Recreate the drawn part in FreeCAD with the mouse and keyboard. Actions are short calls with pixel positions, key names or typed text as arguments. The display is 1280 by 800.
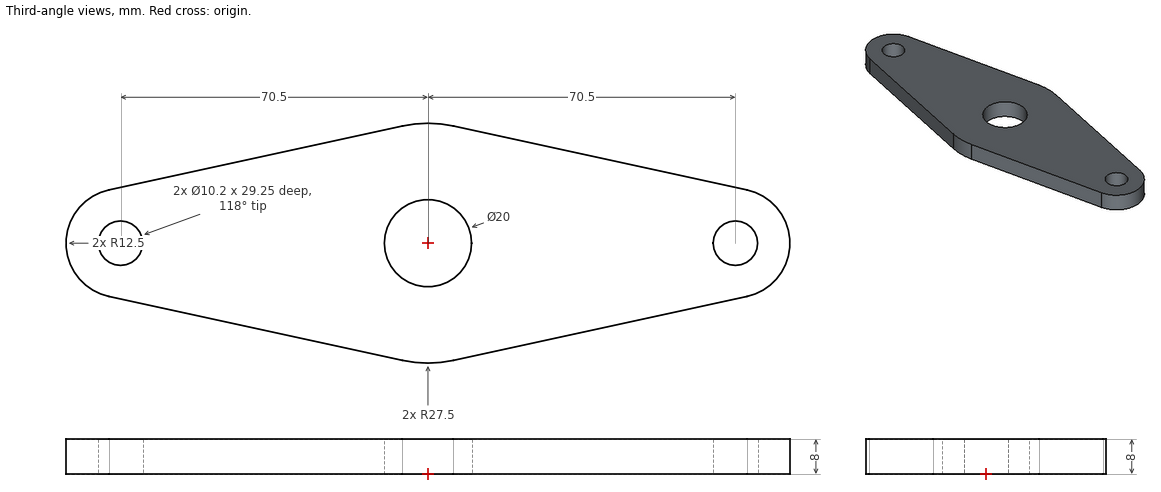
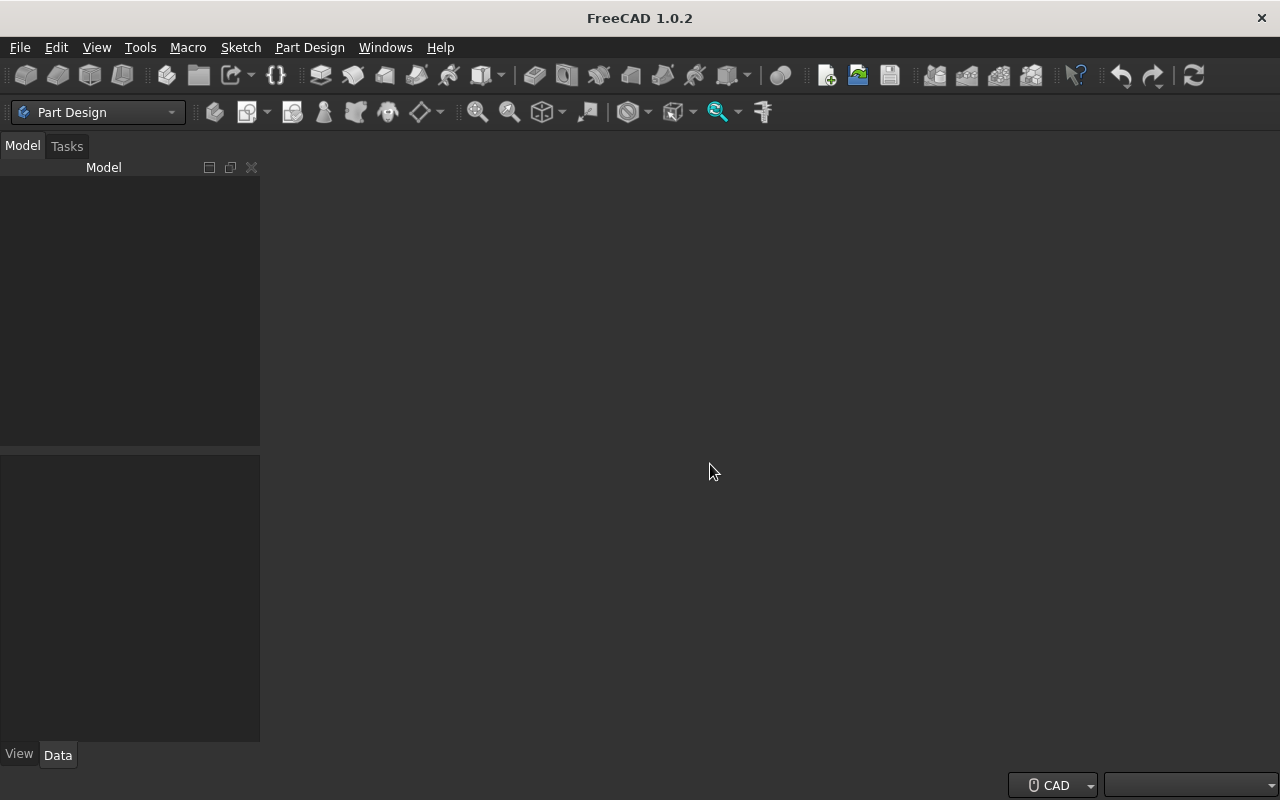
click(826, 76)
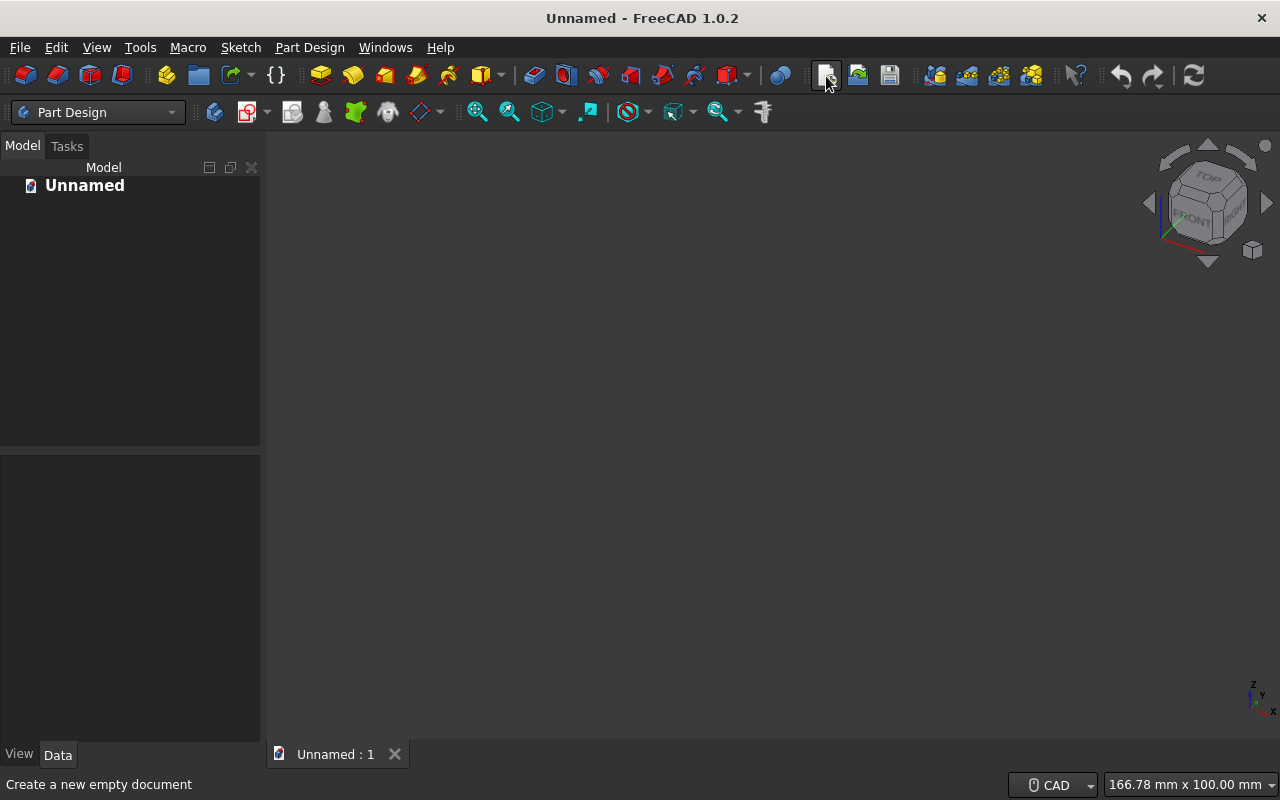
click(248, 112)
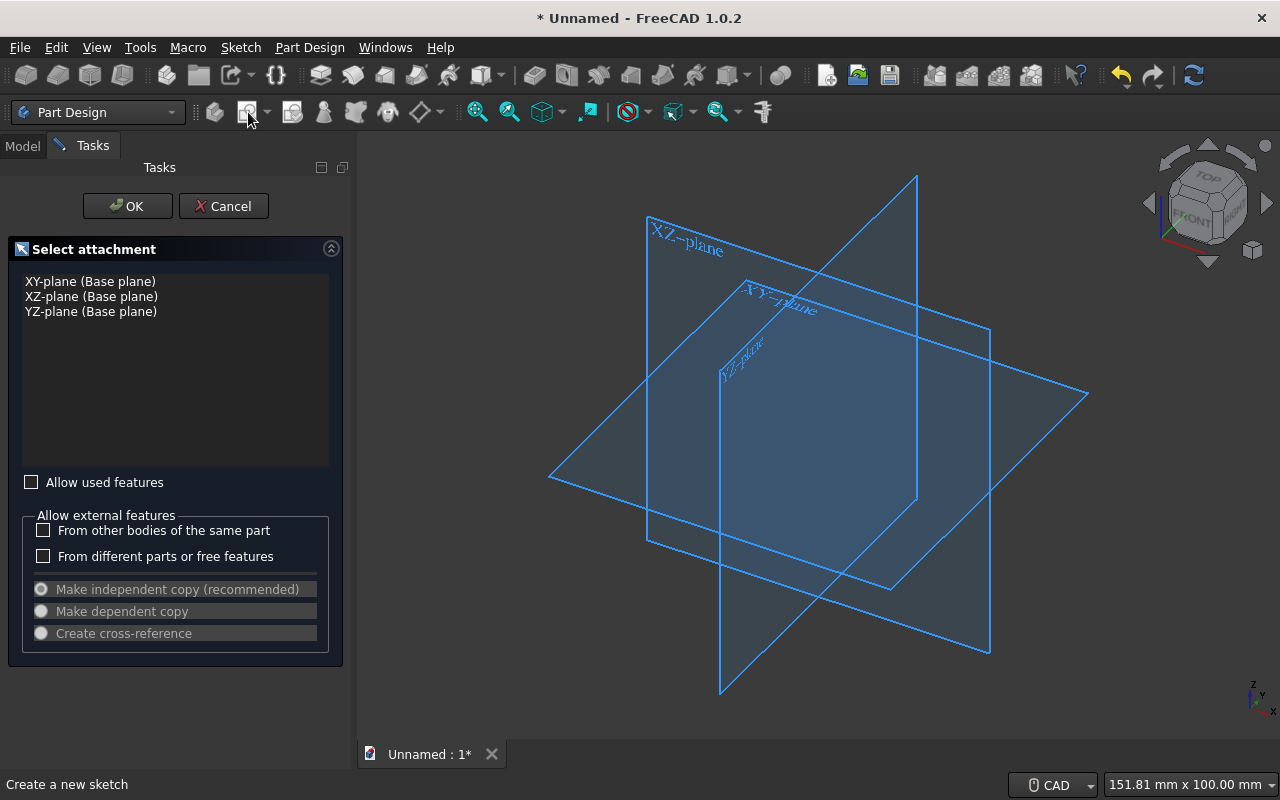
click(82, 282)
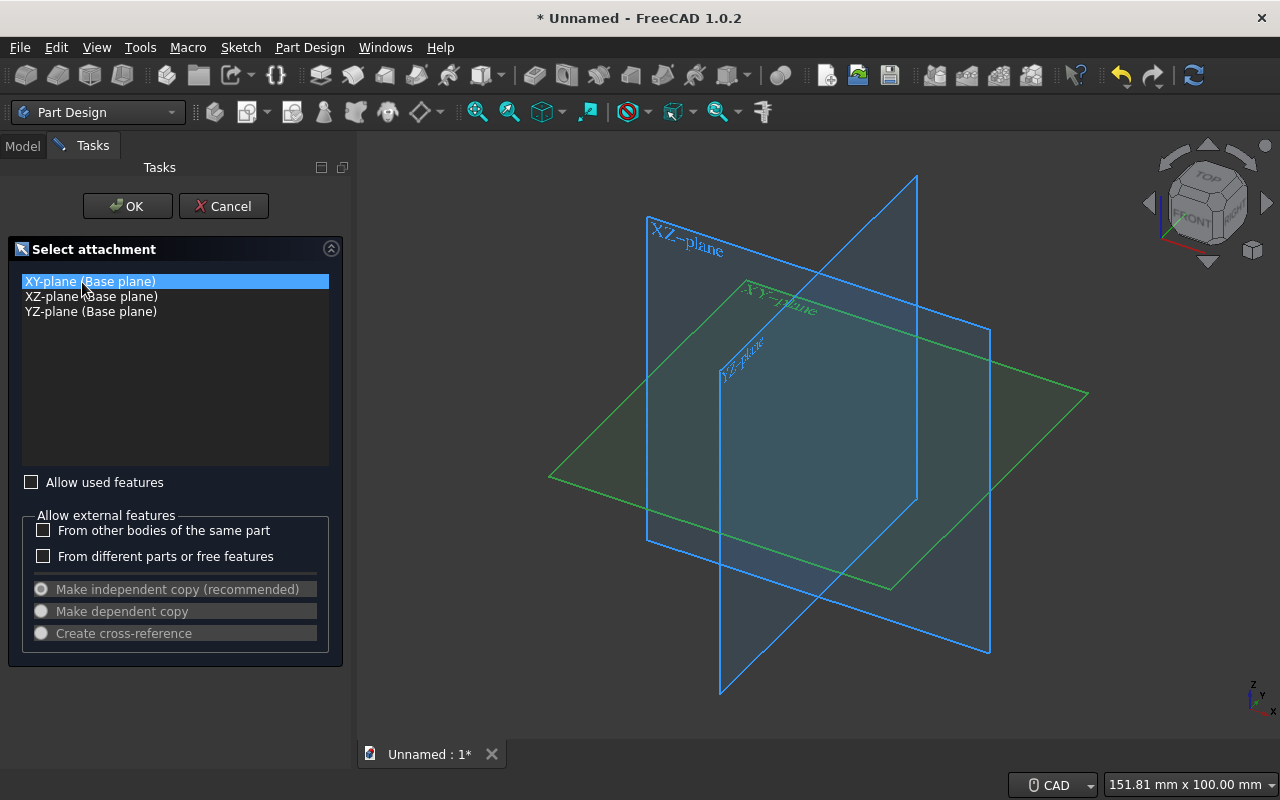
click(128, 206)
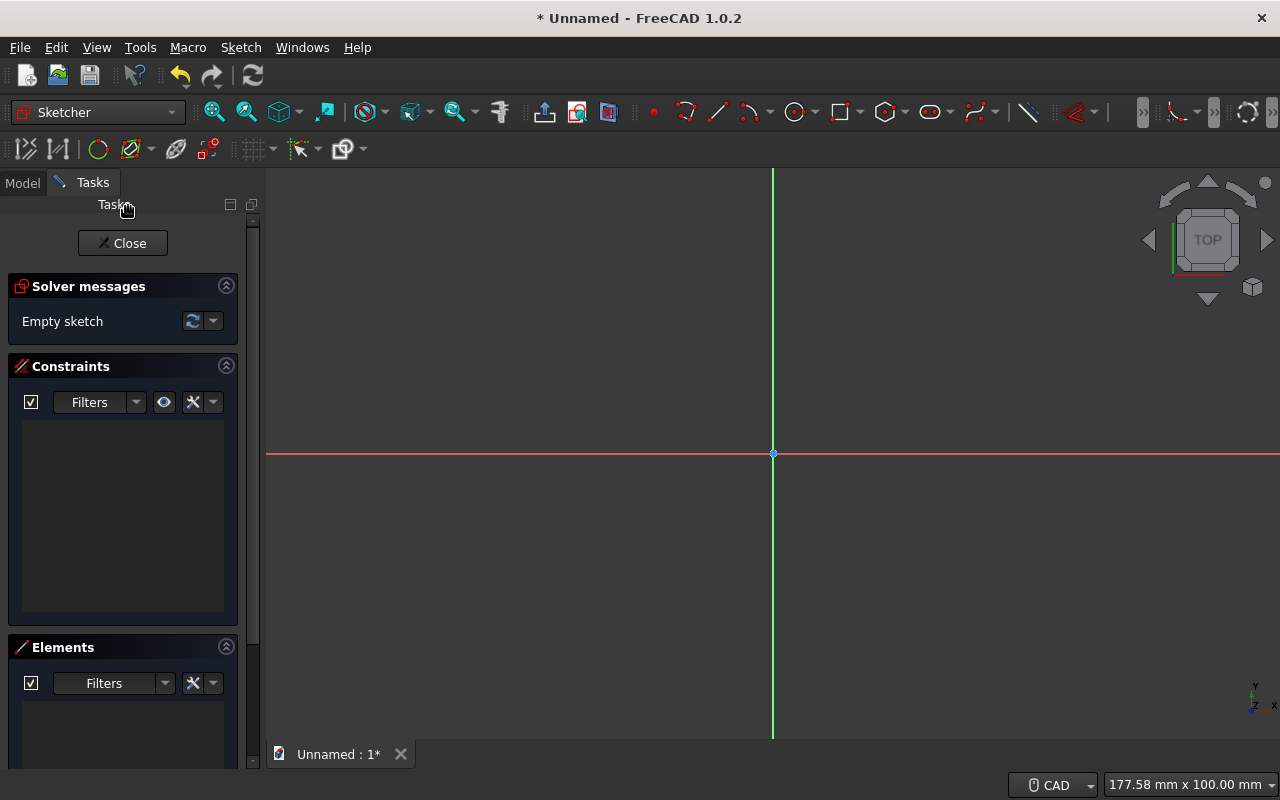
scroll(565, 453, down, 2)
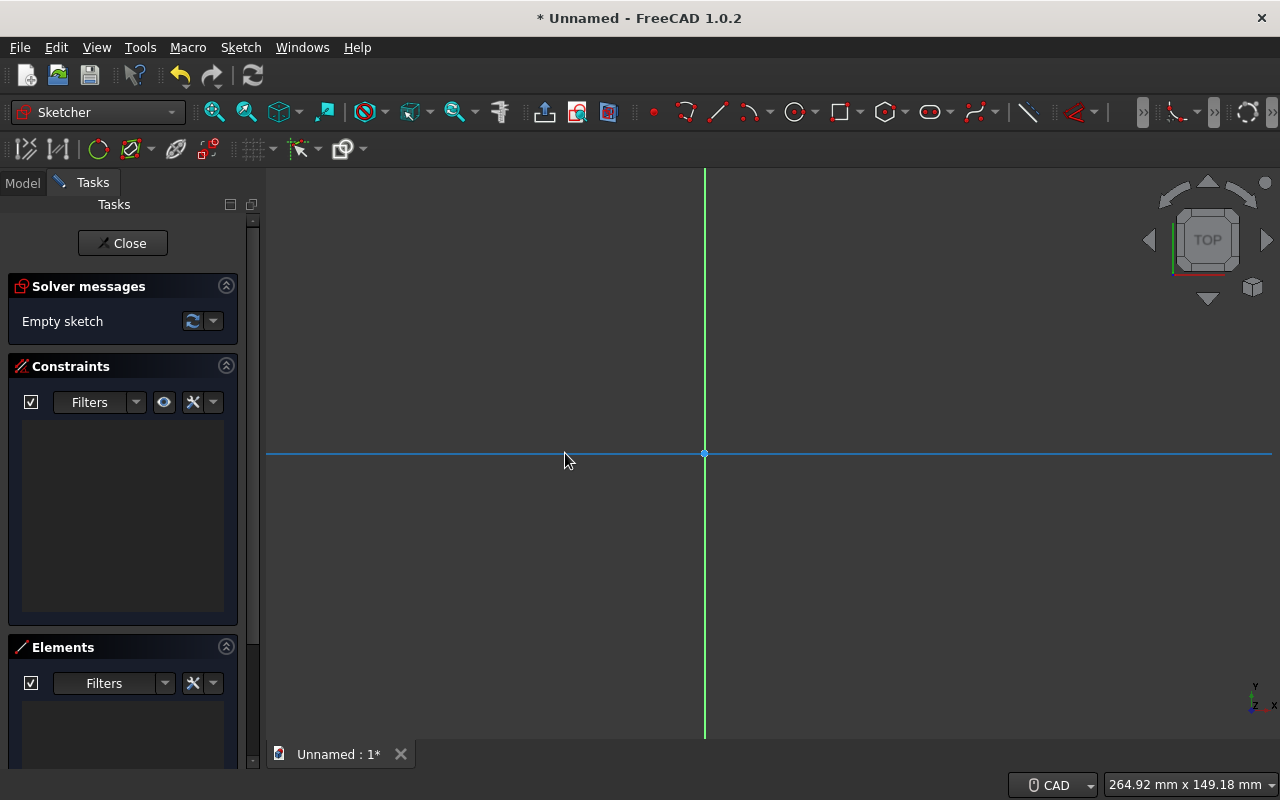
click(718, 112)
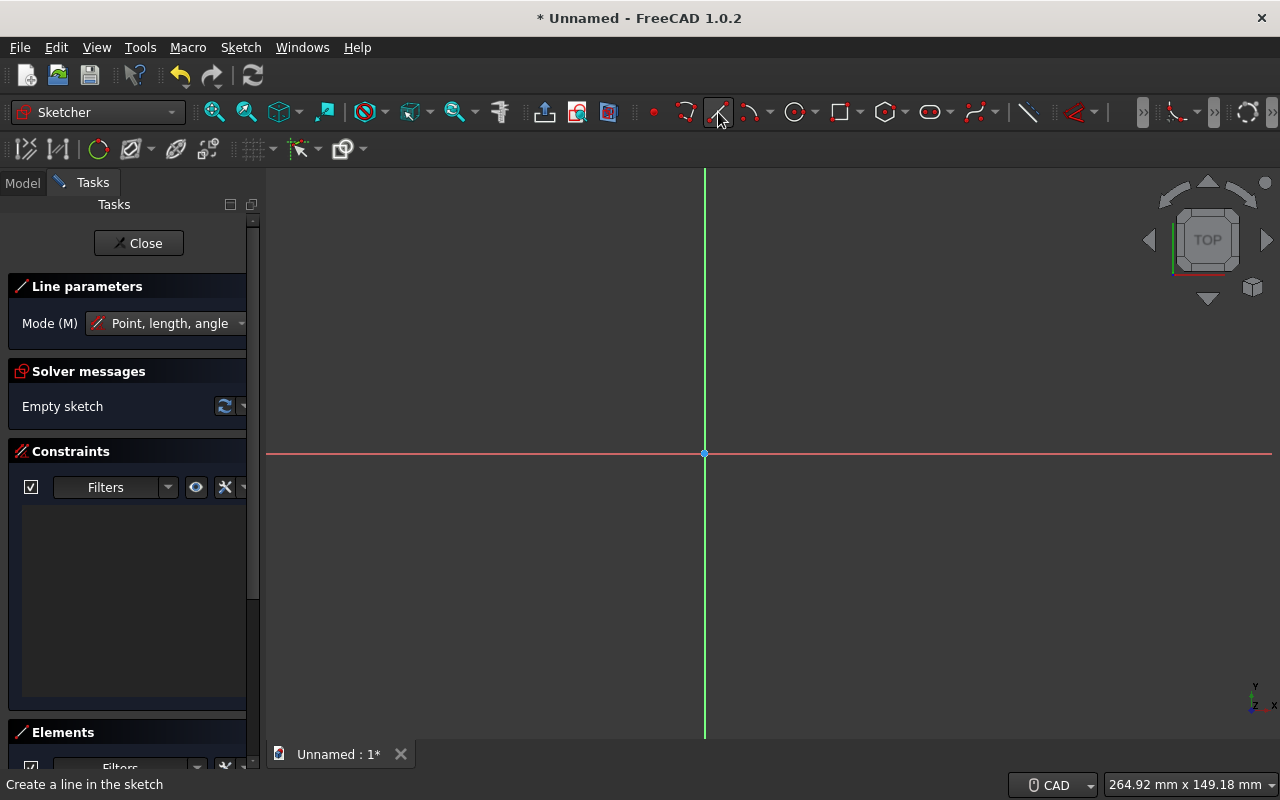
click(682, 351)
click(425, 407)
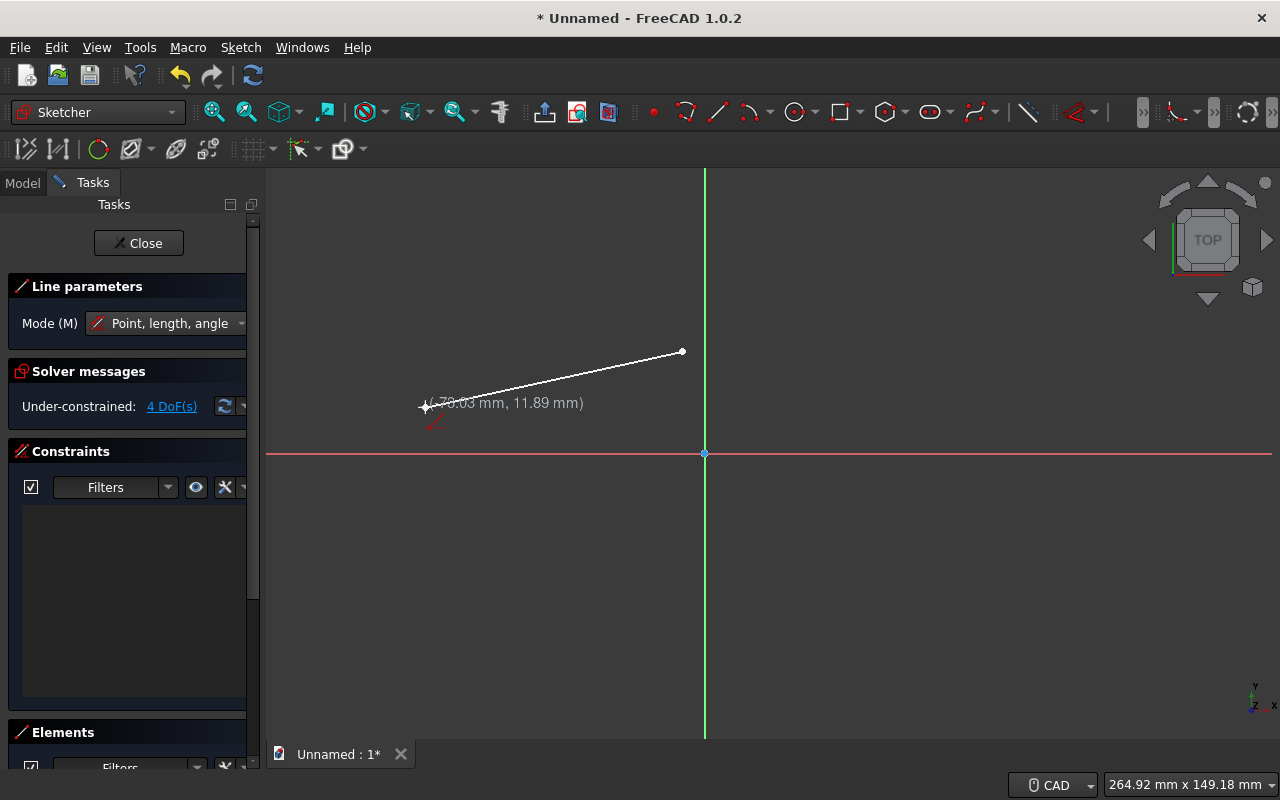
click(425, 500)
click(682, 556)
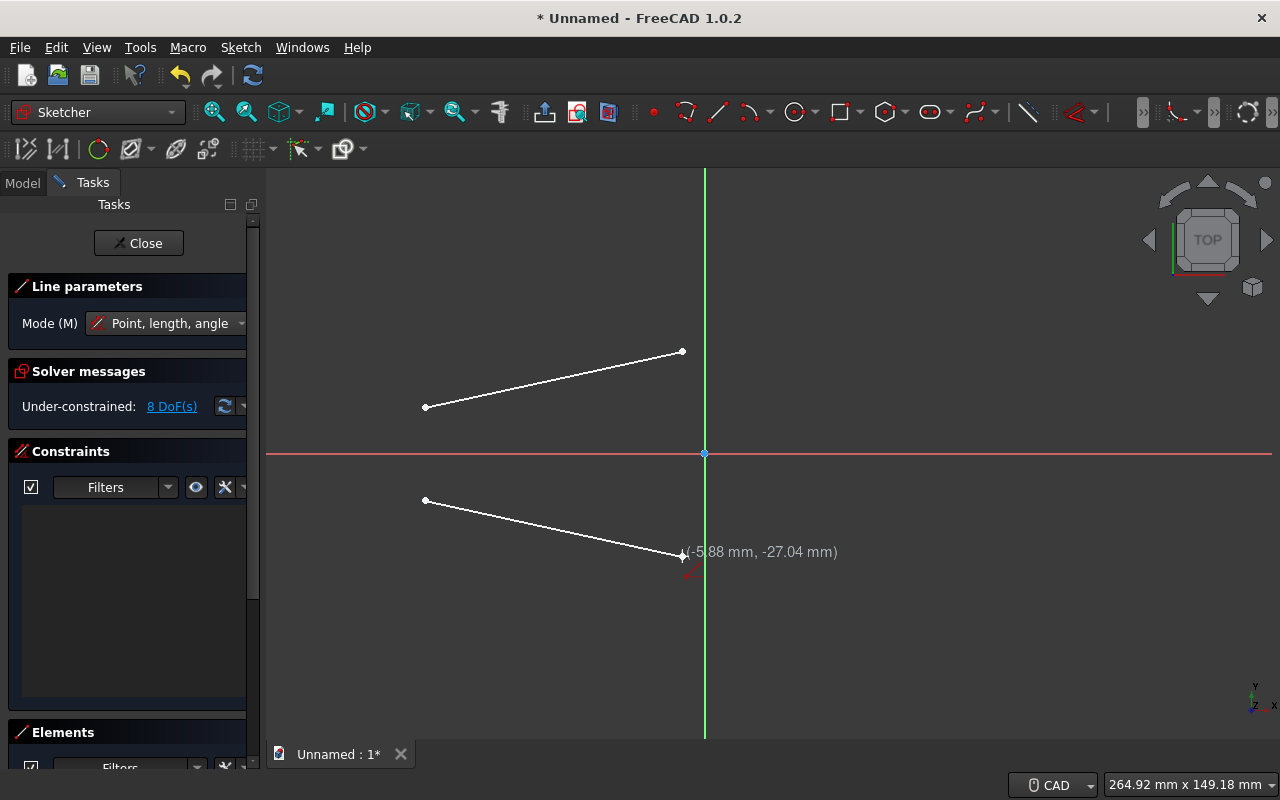
click(727, 556)
click(985, 500)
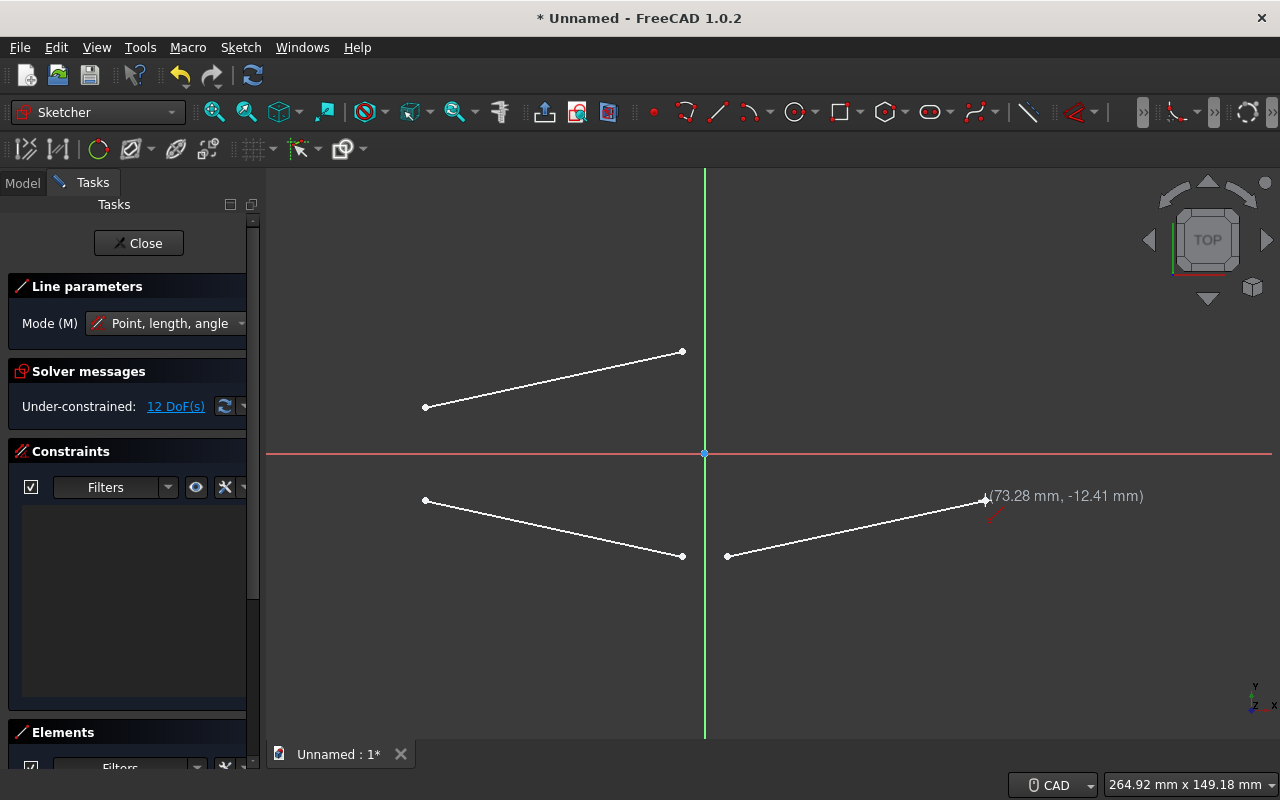
click(985, 407)
click(727, 351)